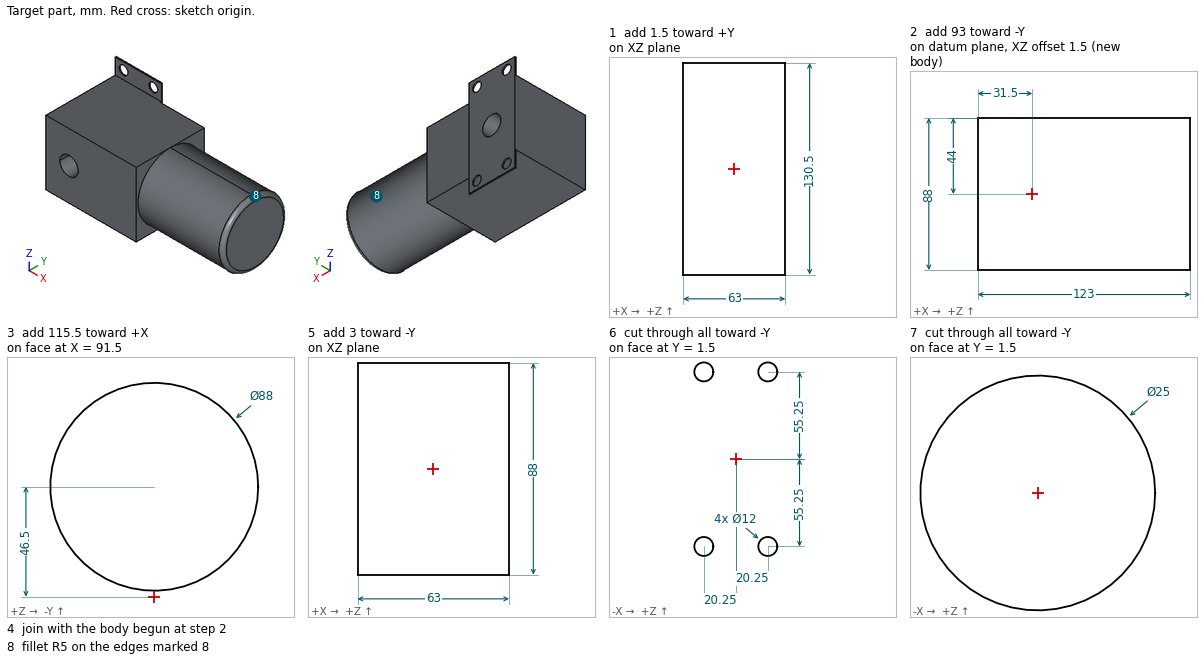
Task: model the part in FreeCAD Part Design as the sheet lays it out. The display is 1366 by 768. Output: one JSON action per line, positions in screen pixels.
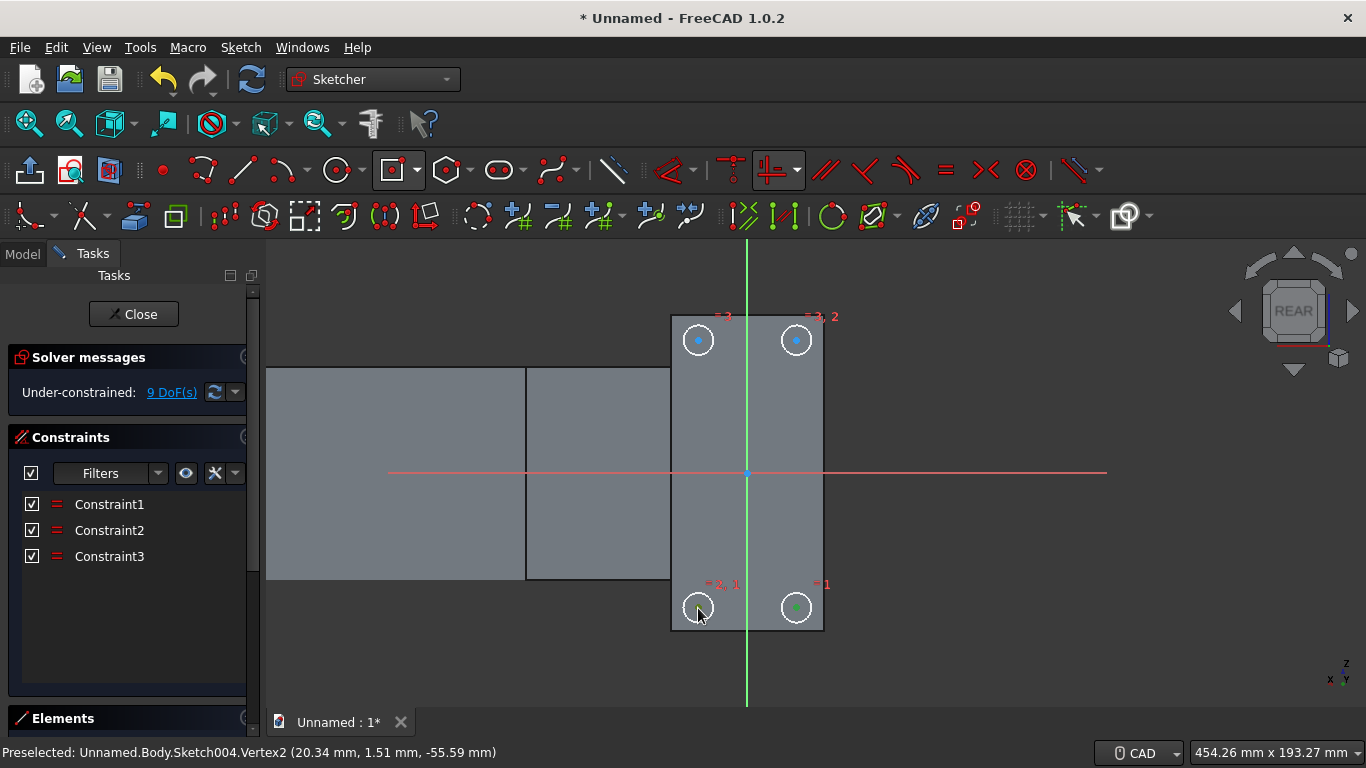
{"action": "key", "text": "h"}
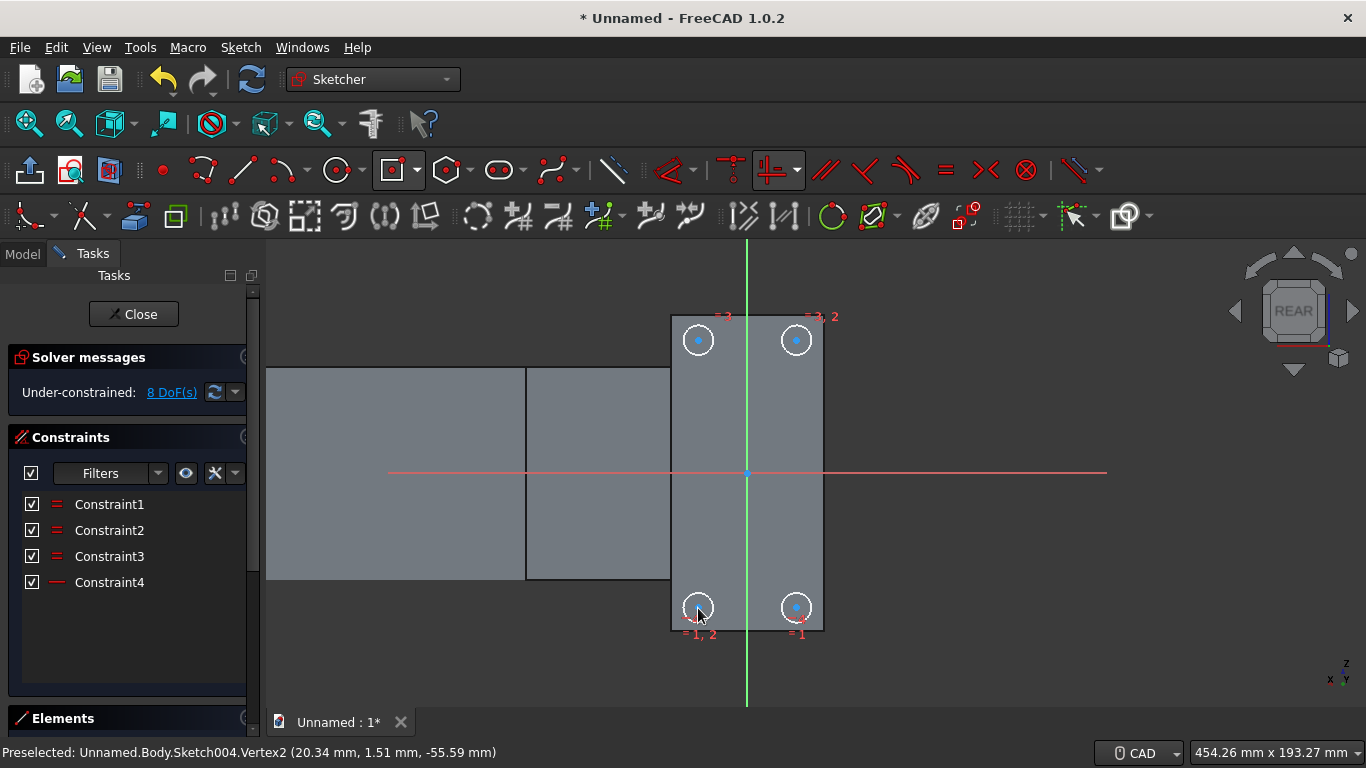
{"action": "left_click", "coordinate": [796, 608]}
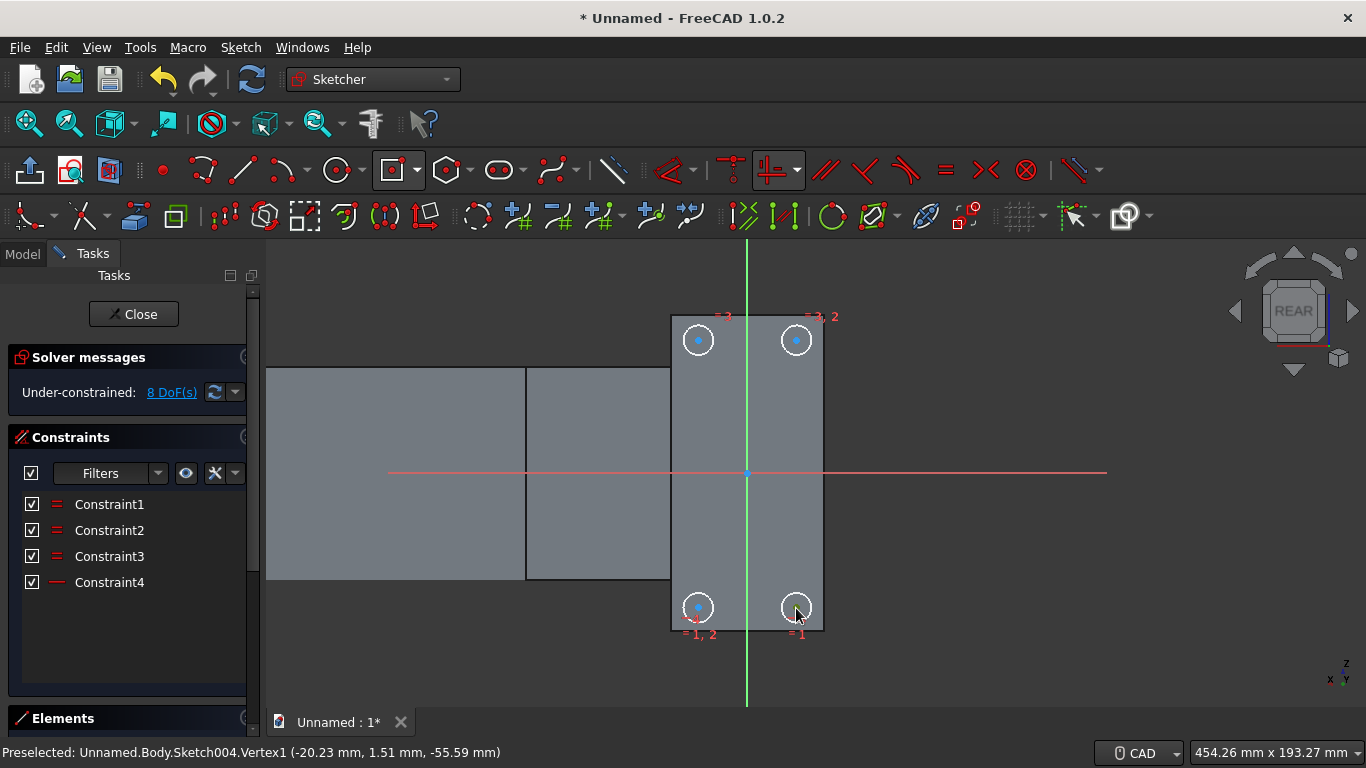
{"action": "left_click", "coordinate": [797, 340]}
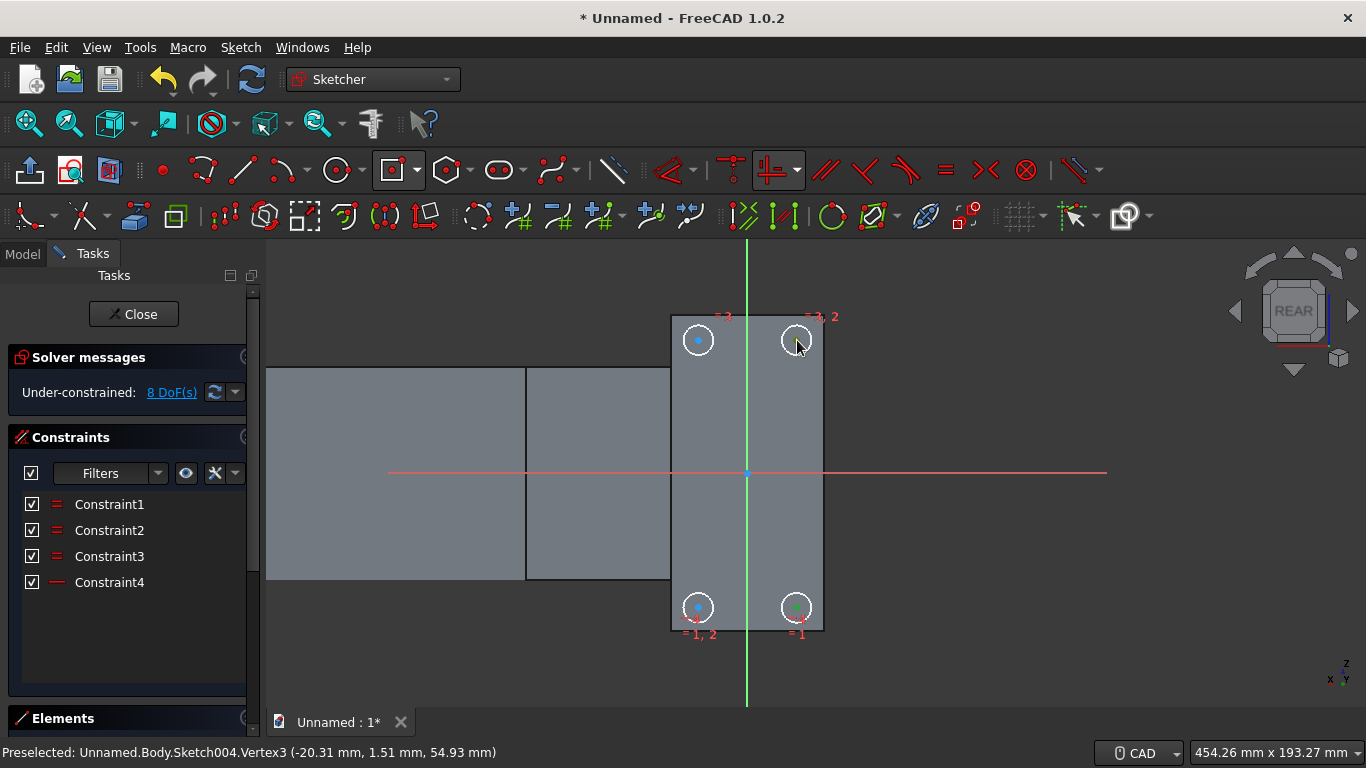
{"action": "key", "text": "v"}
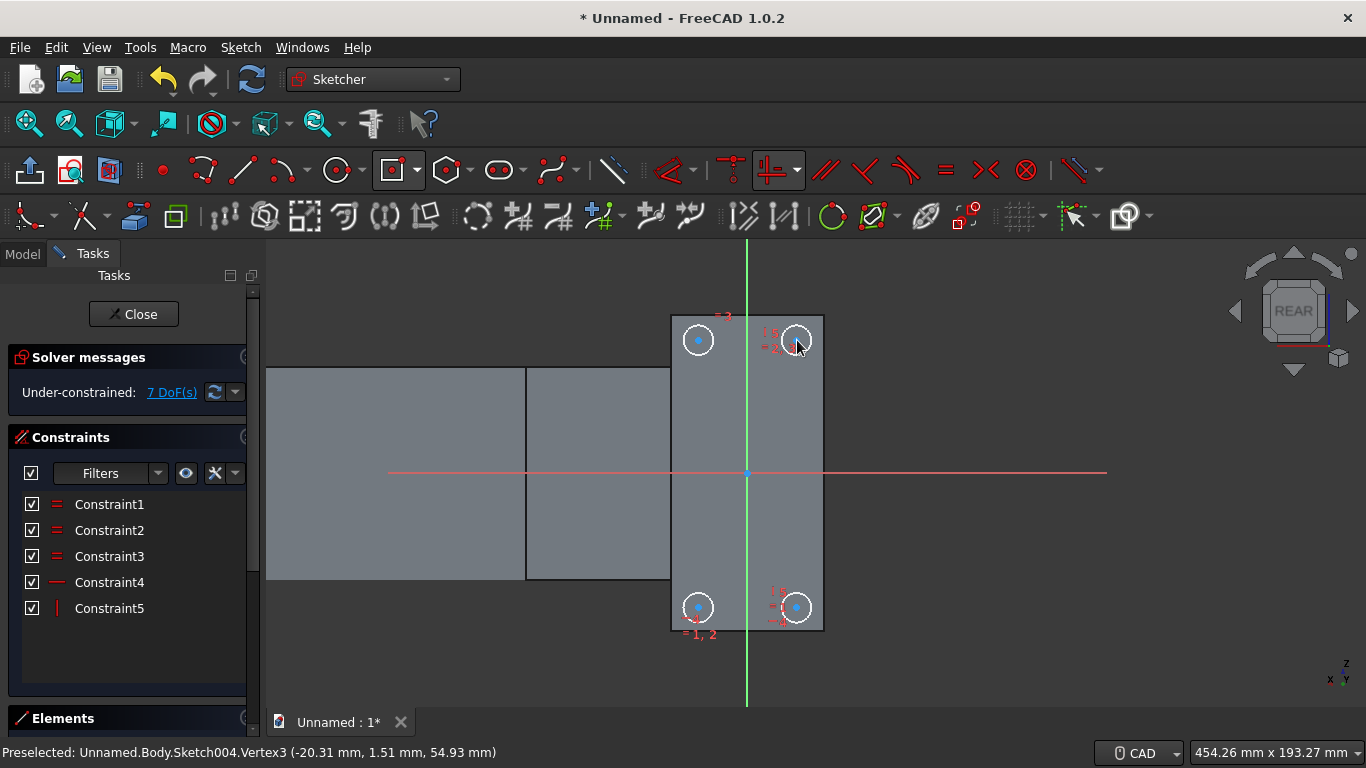
{"action": "left_click", "coordinate": [698, 608]}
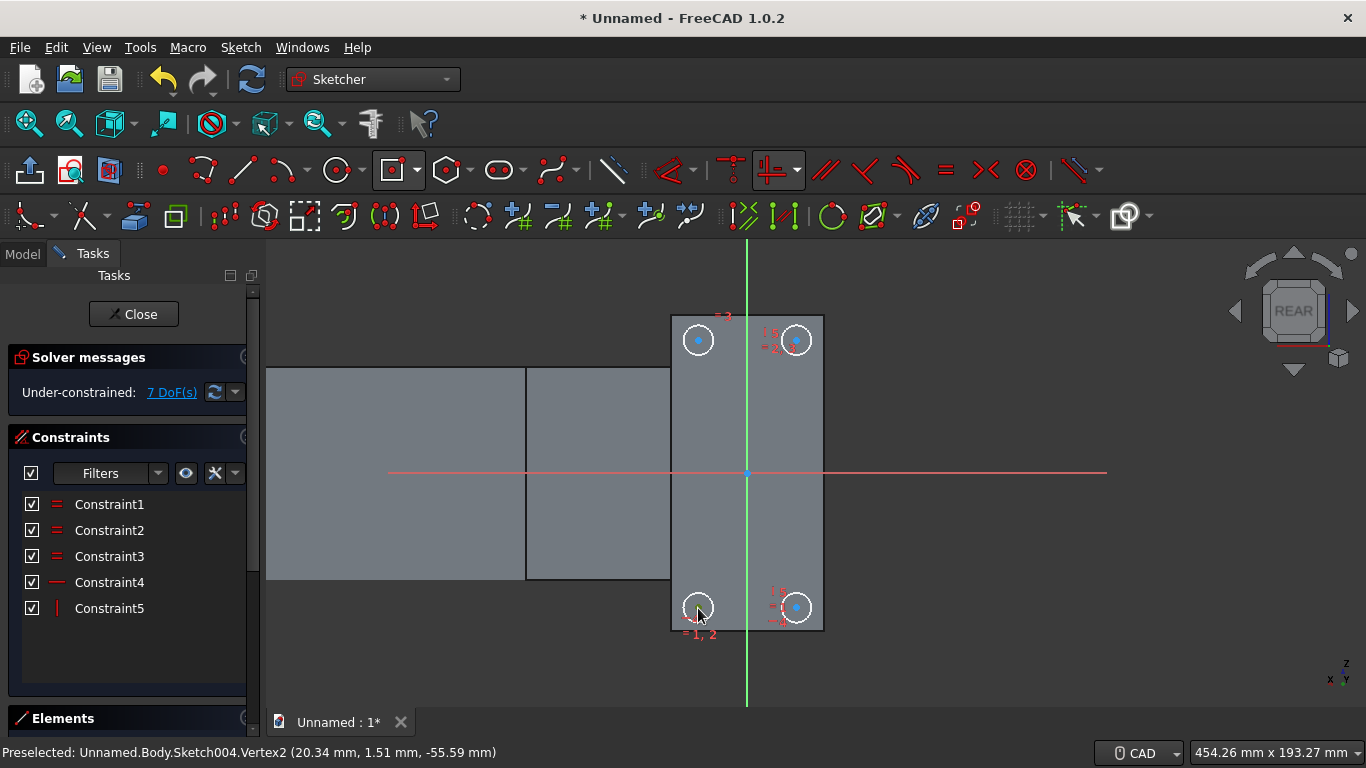
{"action": "left_click", "coordinate": [698, 340]}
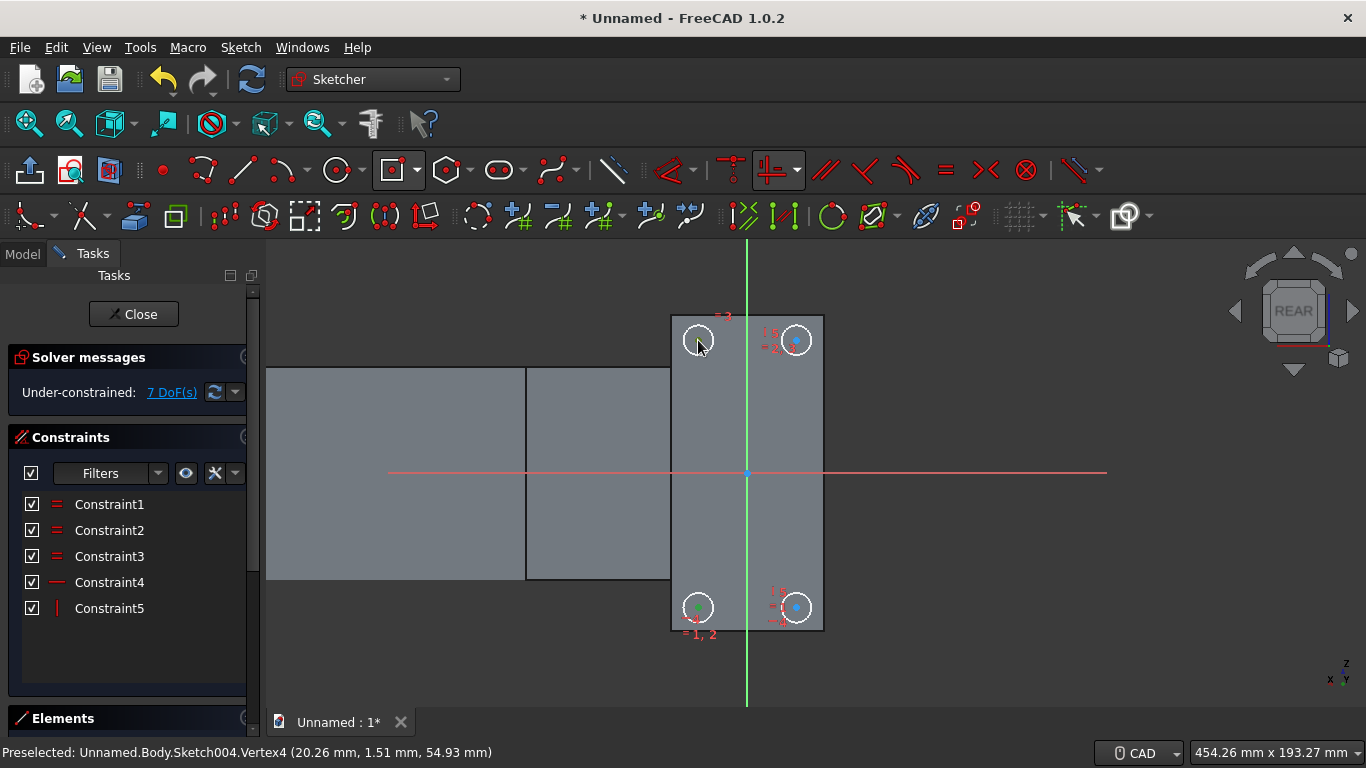
{"action": "left_click", "coordinate": [800, 170]}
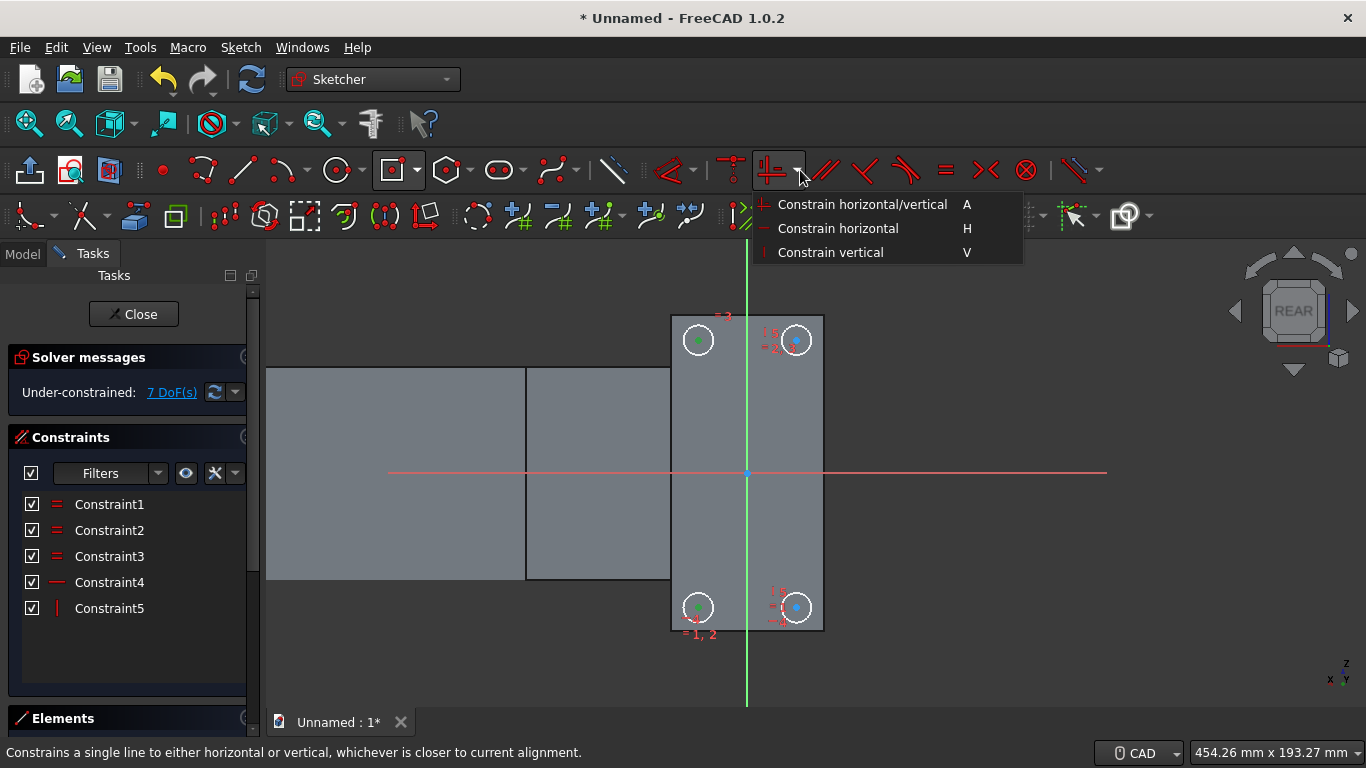
{"action": "left_click", "coordinate": [888, 252]}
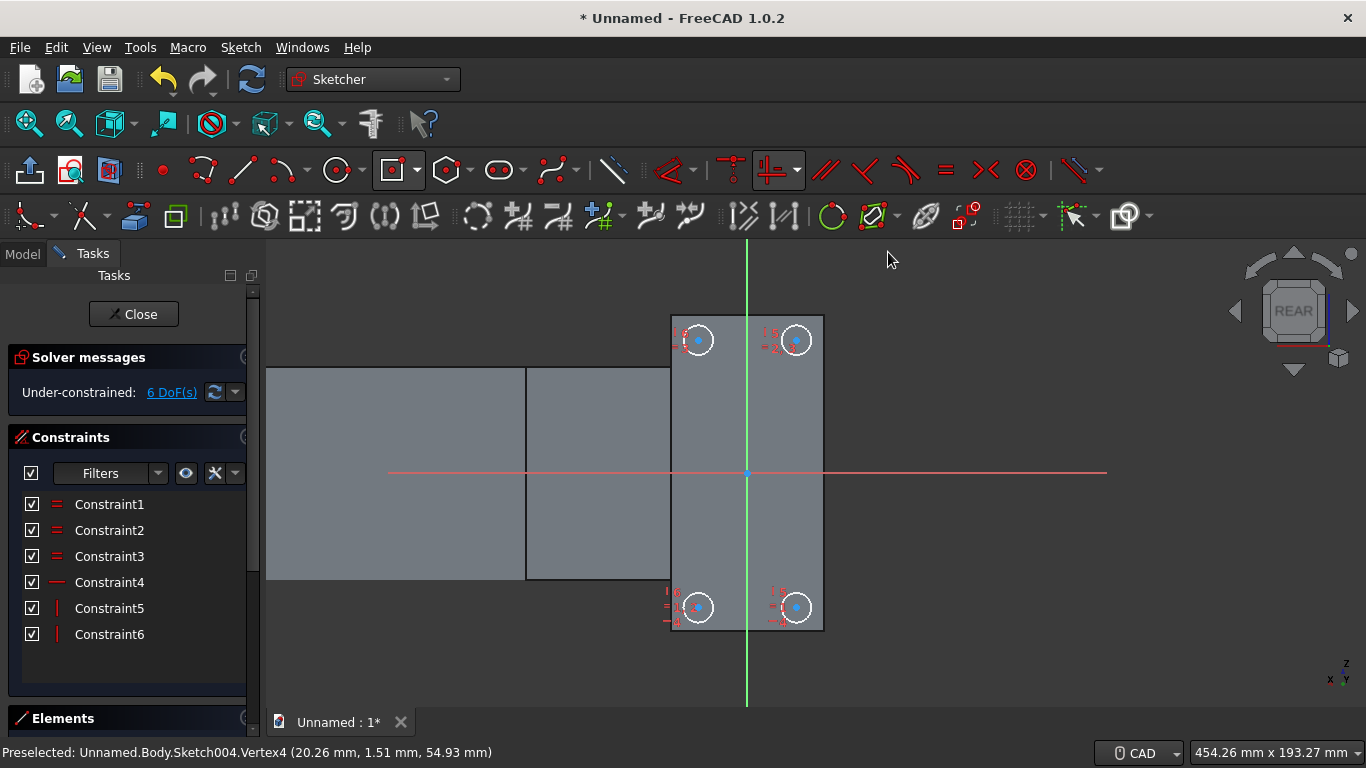
{"action": "left_click", "coordinate": [798, 342]}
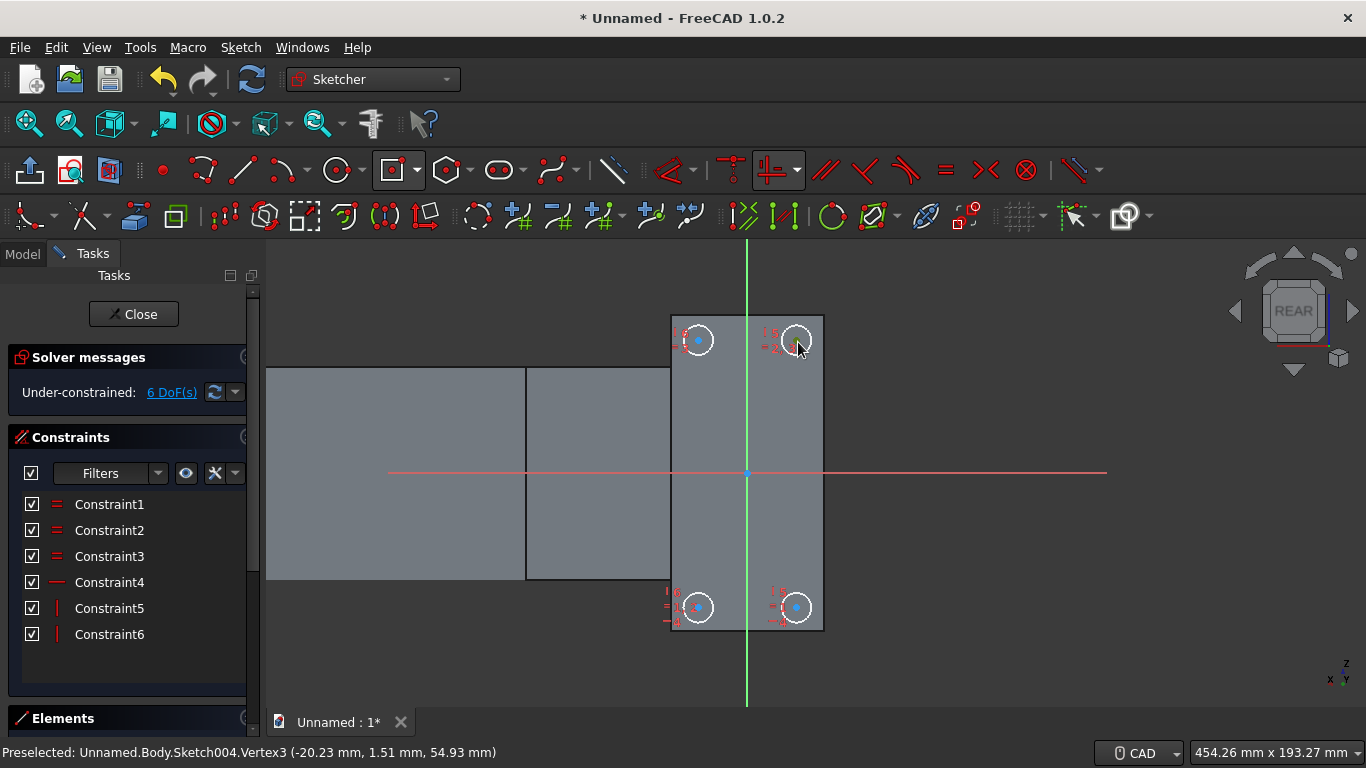
{"action": "left_click", "coordinate": [698, 340]}